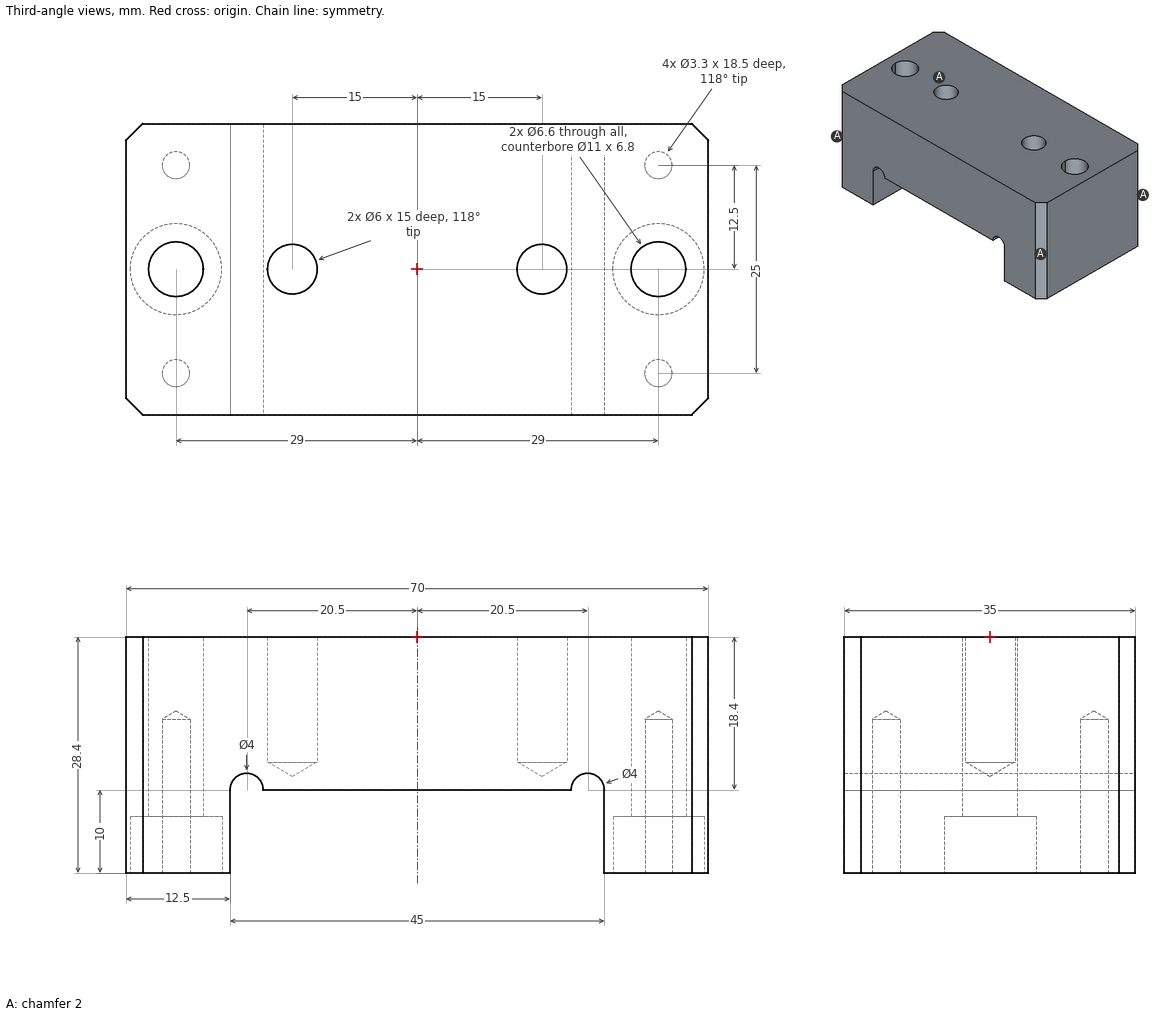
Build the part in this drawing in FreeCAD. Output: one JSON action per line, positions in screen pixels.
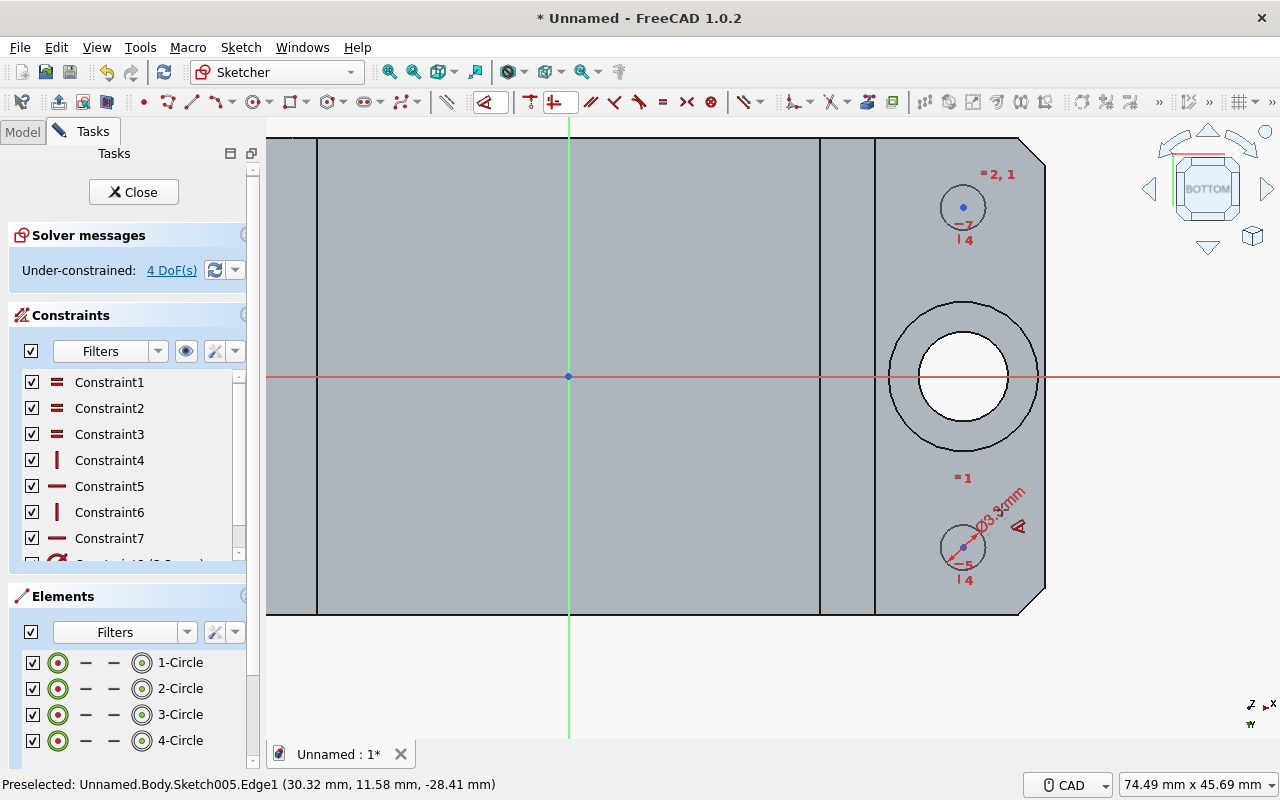
{"action": "left_click", "coordinate": [963, 548]}
{"action": "left_click", "coordinate": [766, 582]}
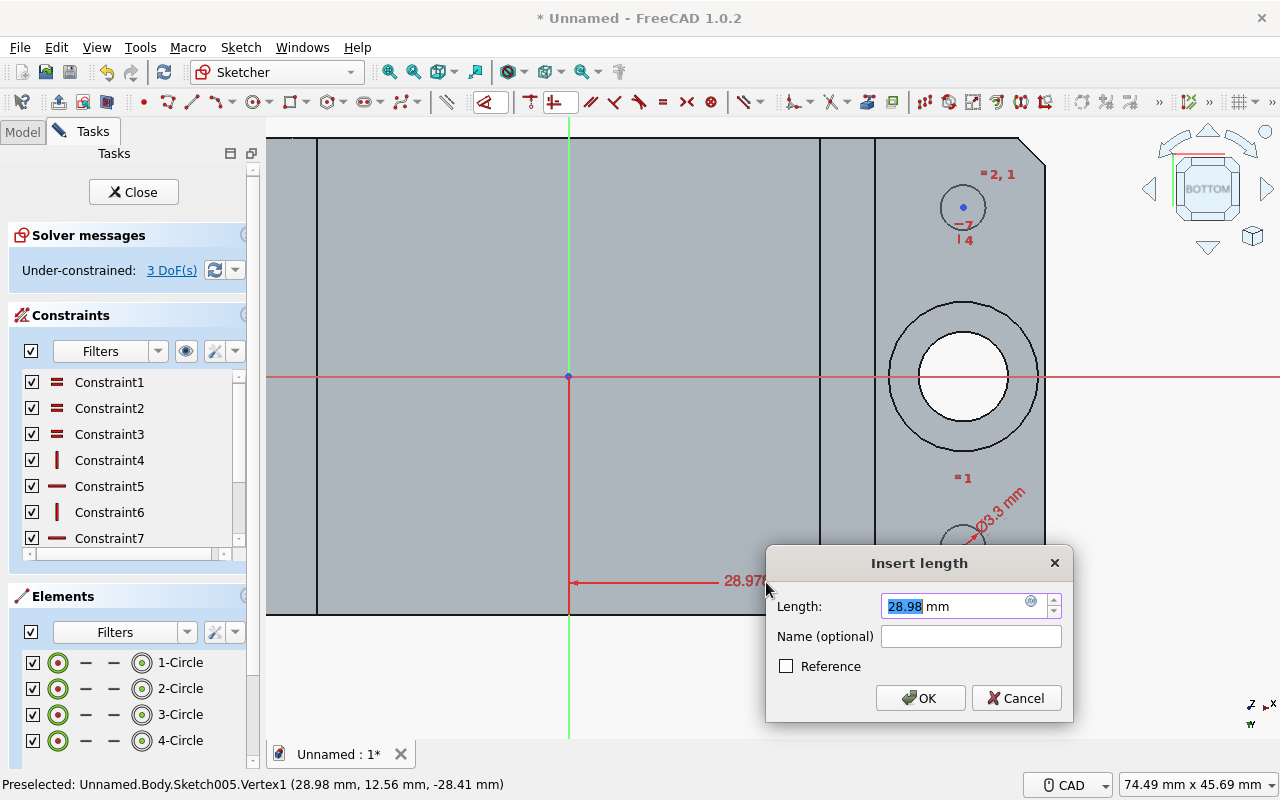
{"action": "type", "text": "29"}
{"action": "key", "text": "Return"}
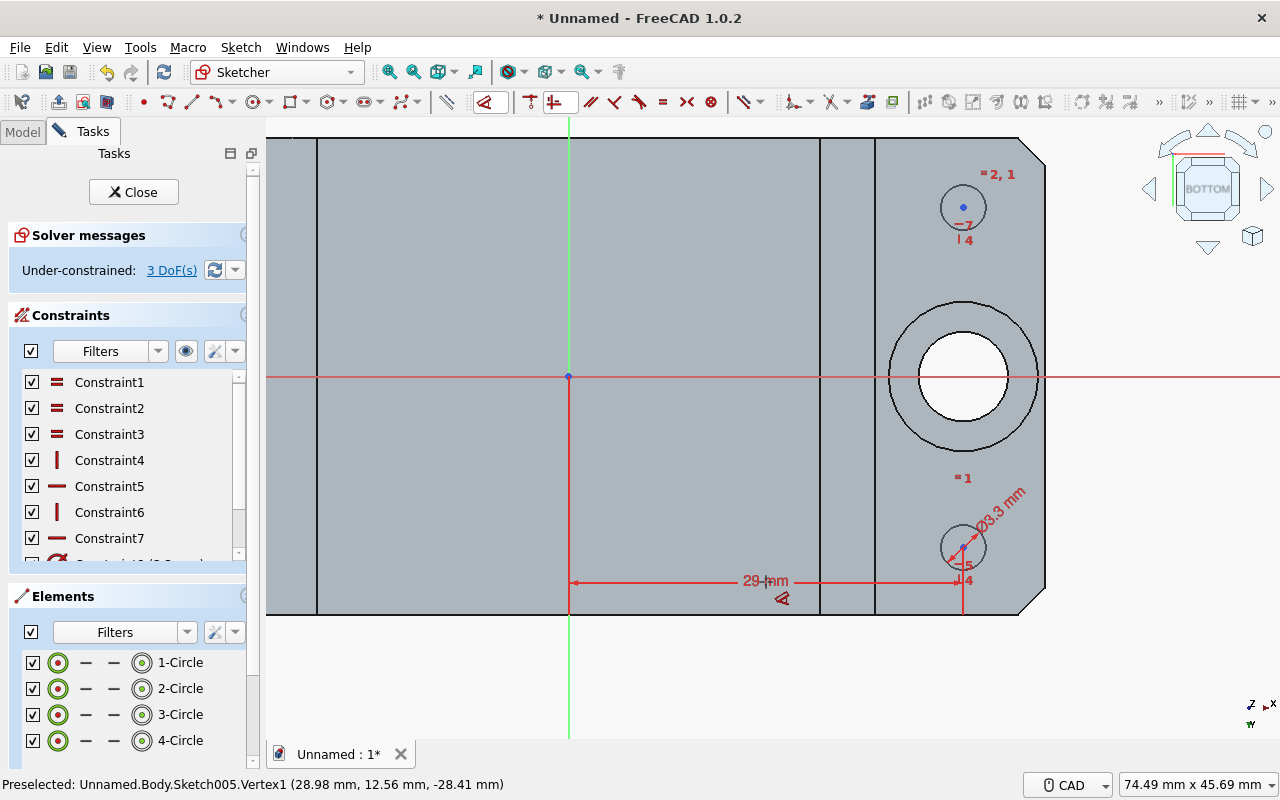
{"action": "scroll", "coordinate": [981, 533], "scroll_direction": "down", "scroll_amount": 2}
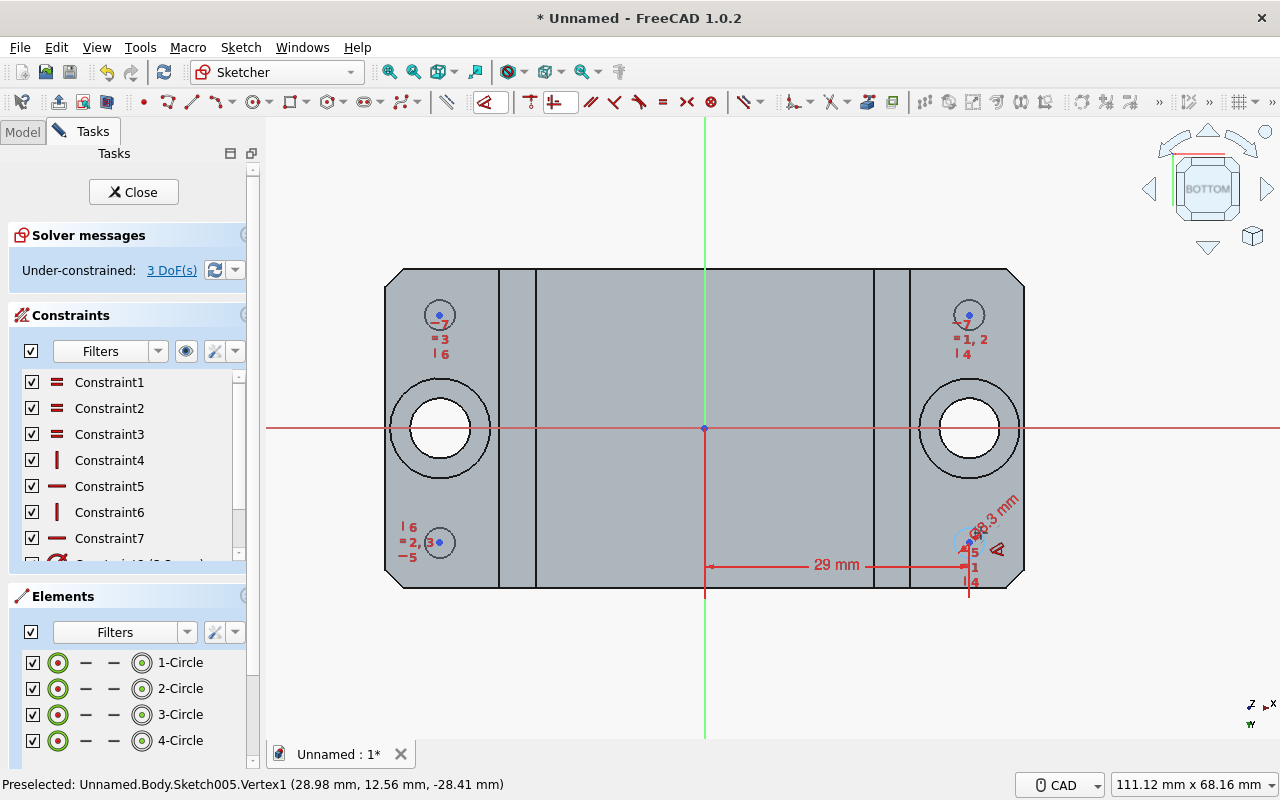
{"action": "left_click", "coordinate": [440, 543]}
{"action": "left_click", "coordinate": [572, 577]}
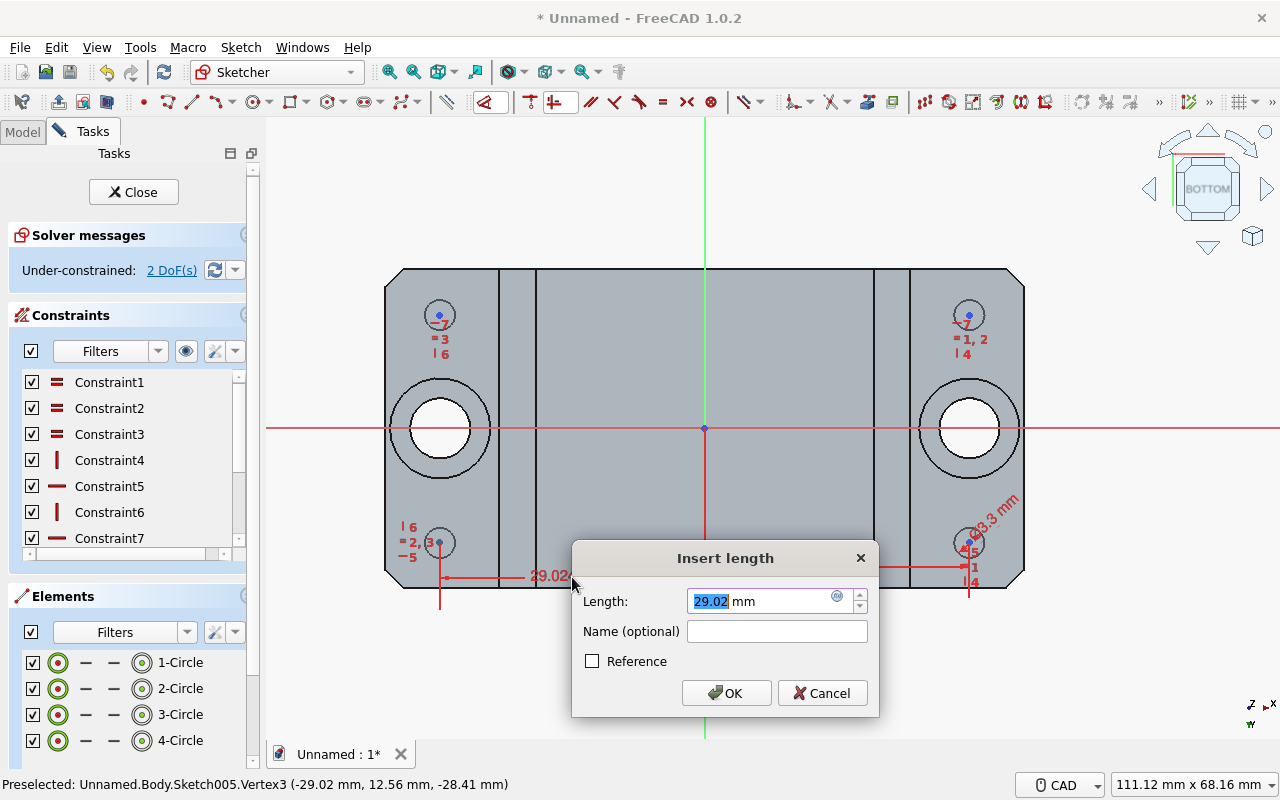
{"action": "type", "text": "29"}
{"action": "key", "text": "Return"}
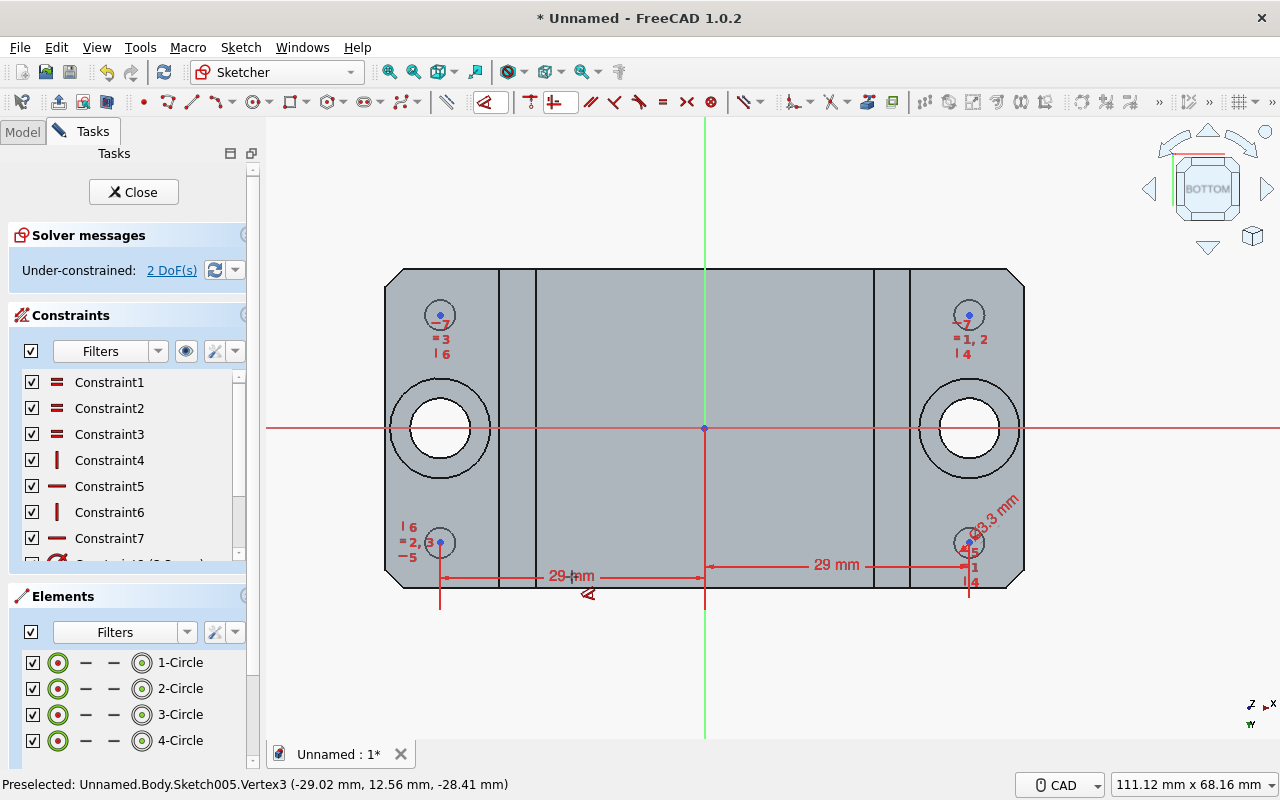
{"action": "left_click", "coordinate": [969, 543]}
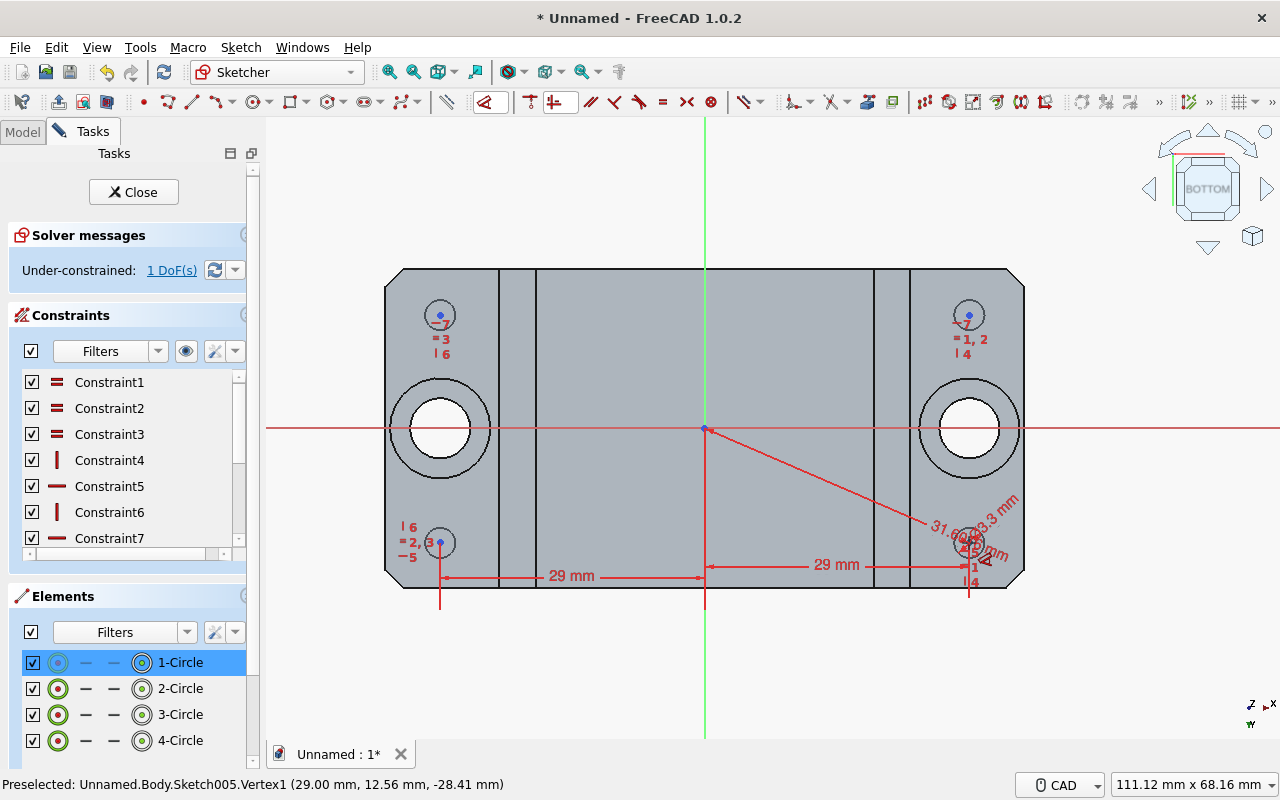
{"action": "left_click", "coordinate": [969, 315]}
{"action": "left_click", "coordinate": [1003, 377]}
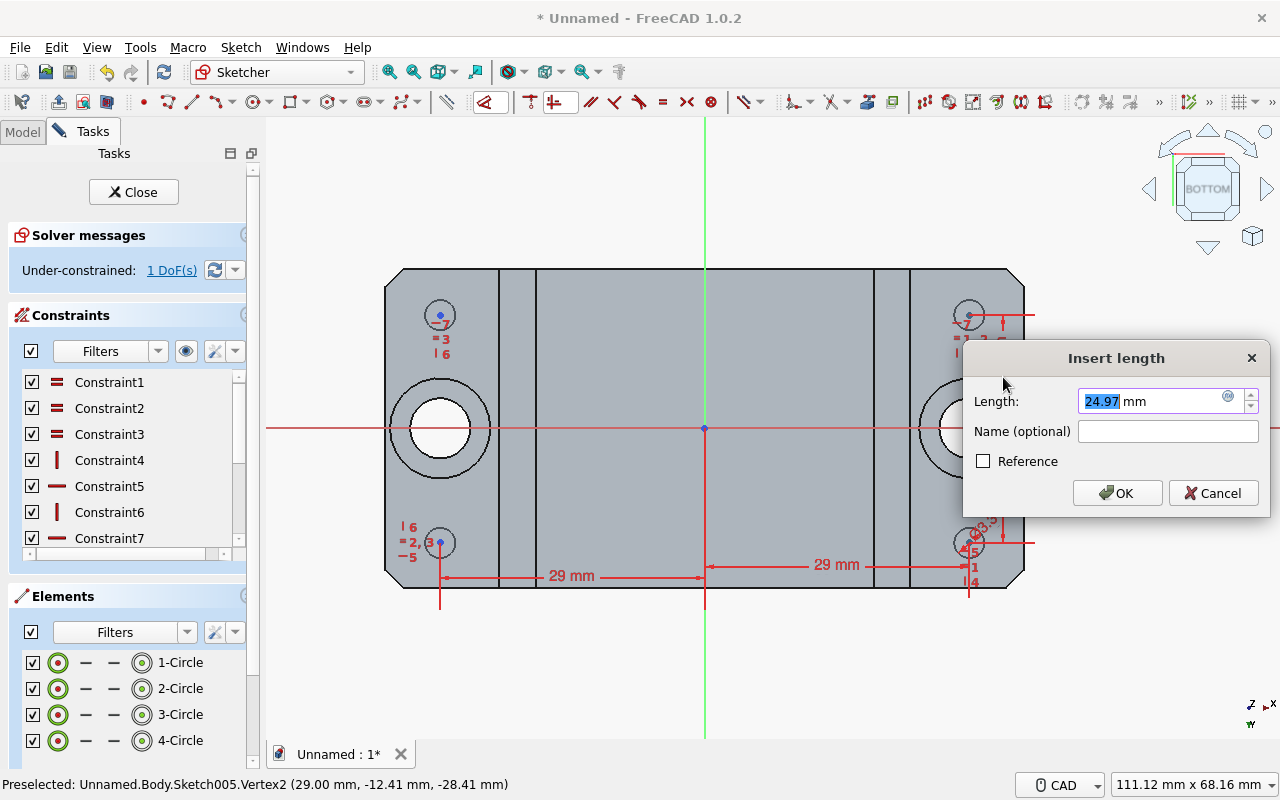
{"action": "type", "text": "25"}
{"action": "key", "text": "Return"}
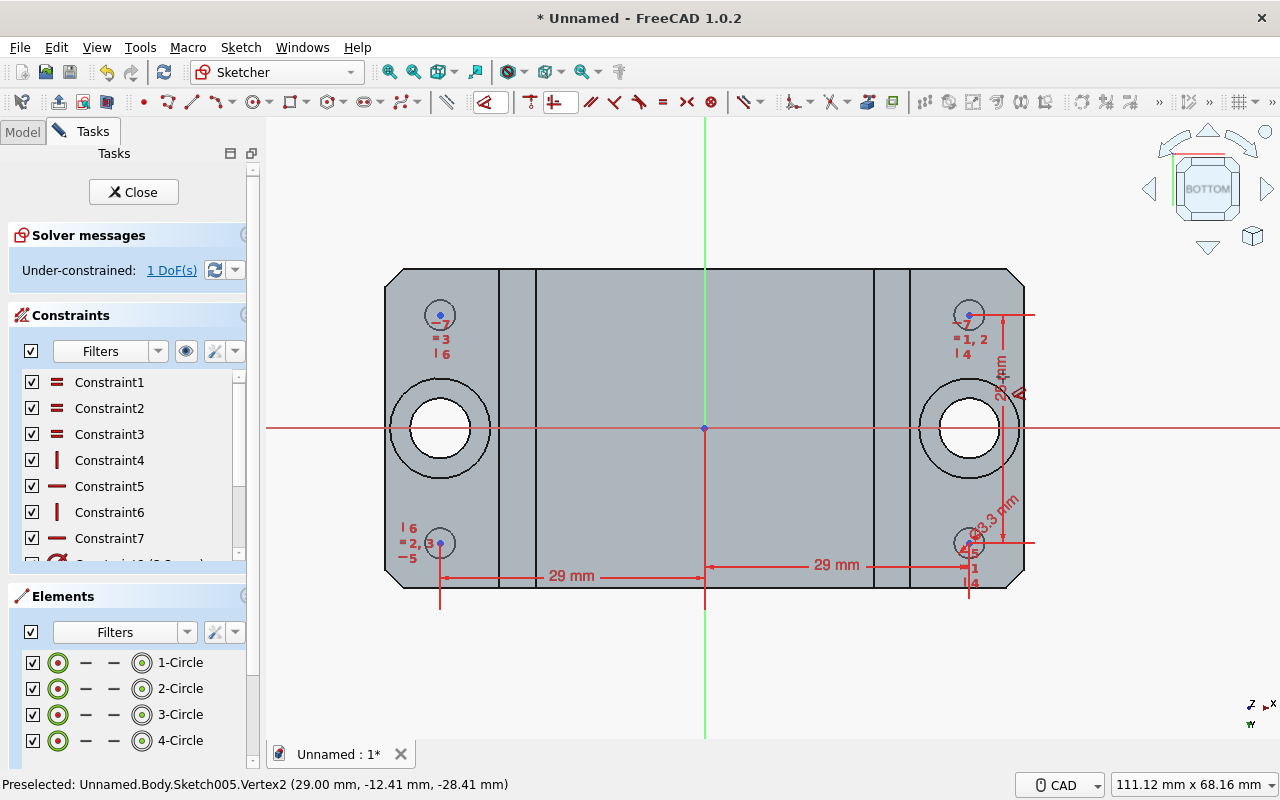
{"action": "left_click", "coordinate": [969, 543]}
{"action": "left_click", "coordinate": [1003, 486]}